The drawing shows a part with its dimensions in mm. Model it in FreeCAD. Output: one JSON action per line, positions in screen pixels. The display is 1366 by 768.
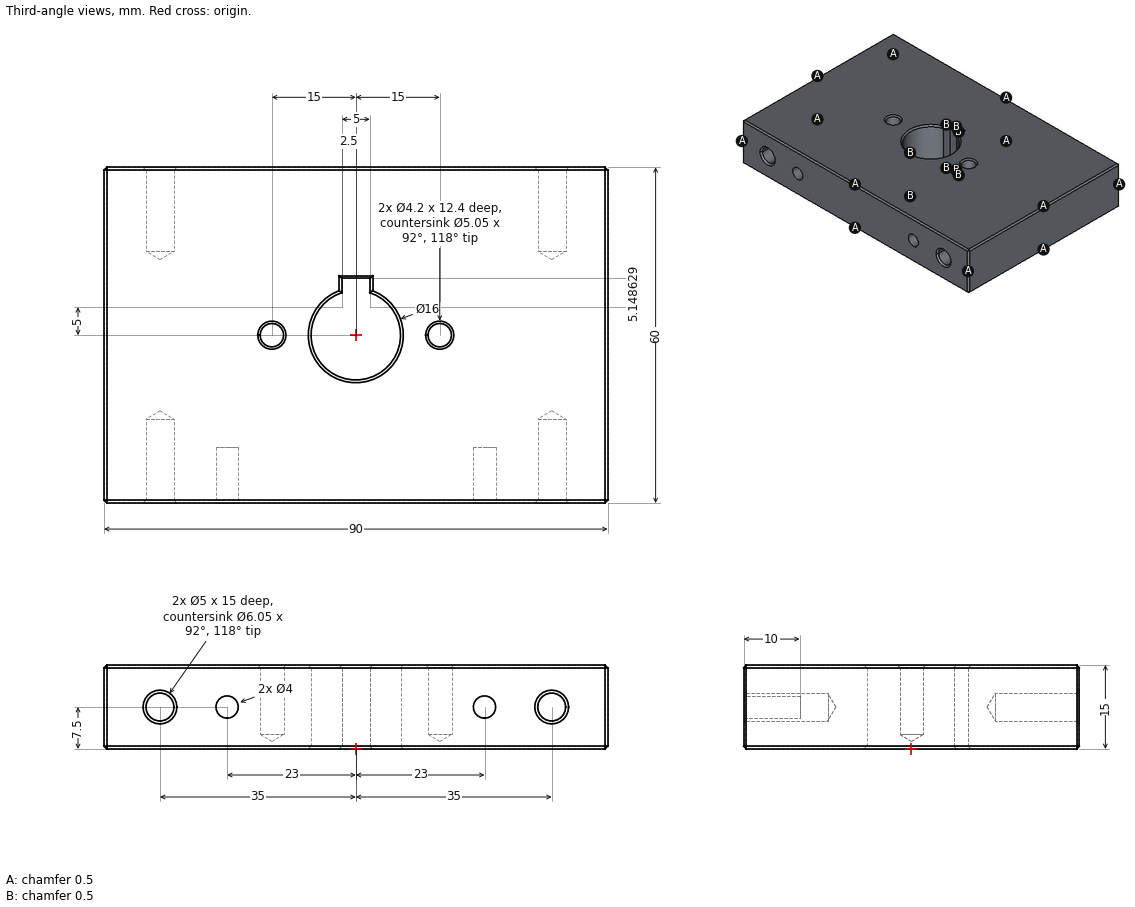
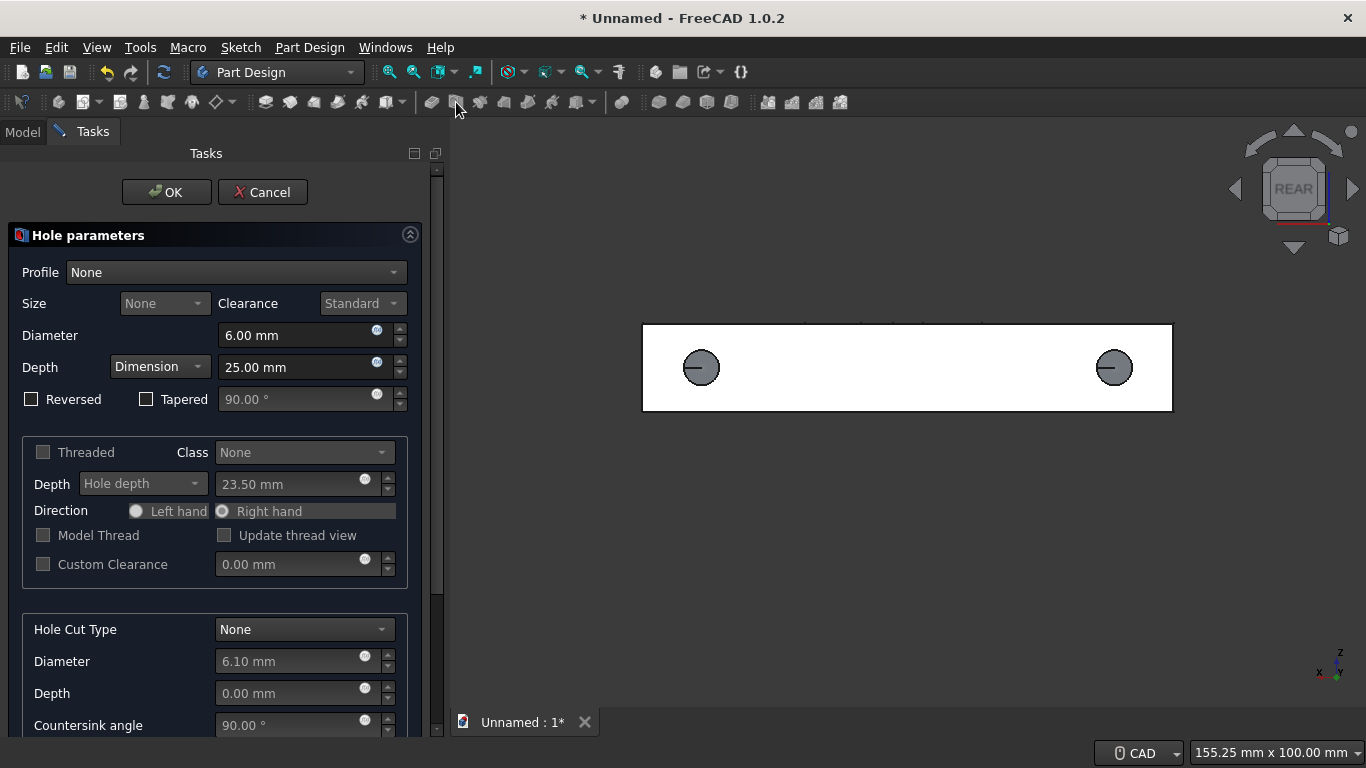
{"action": "triple_click", "coordinate": [305, 335]}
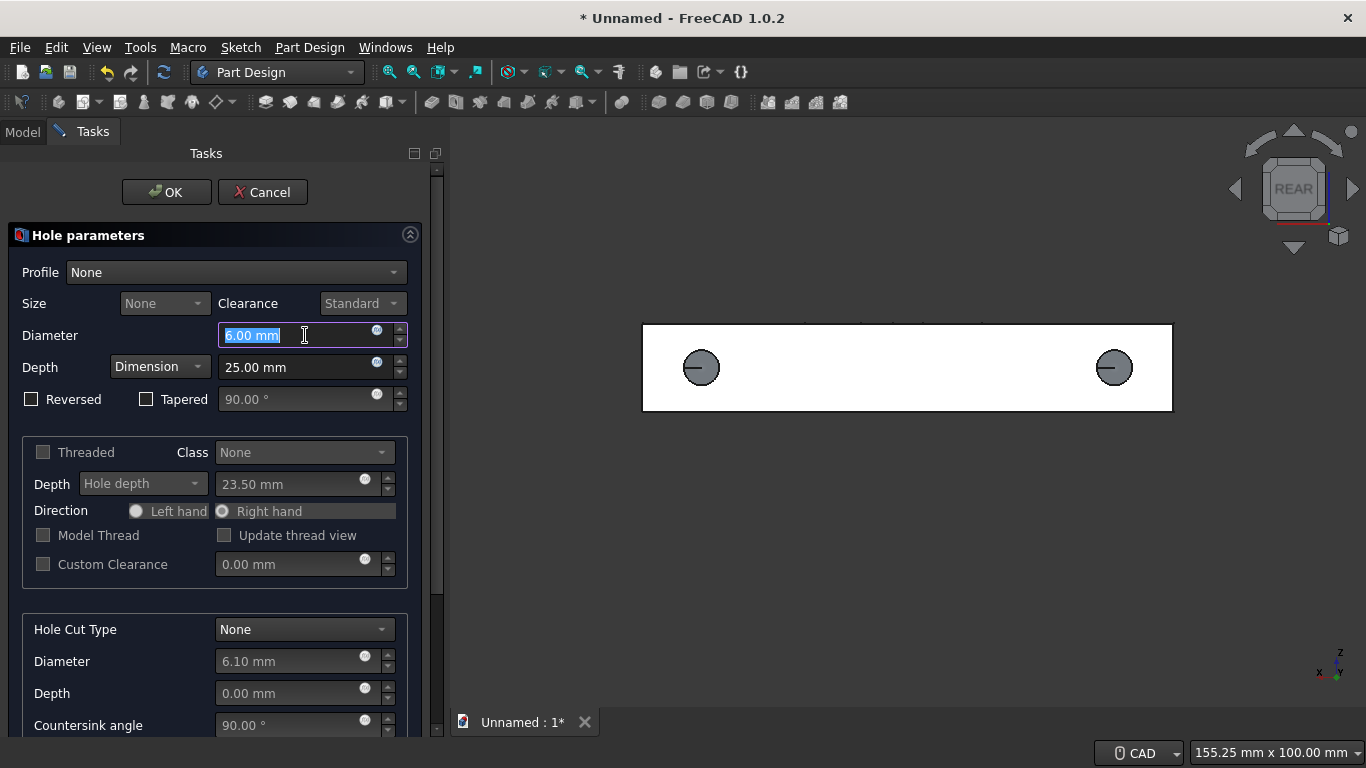
{"action": "type", "text": "5"}
{"action": "key", "text": "Tab"}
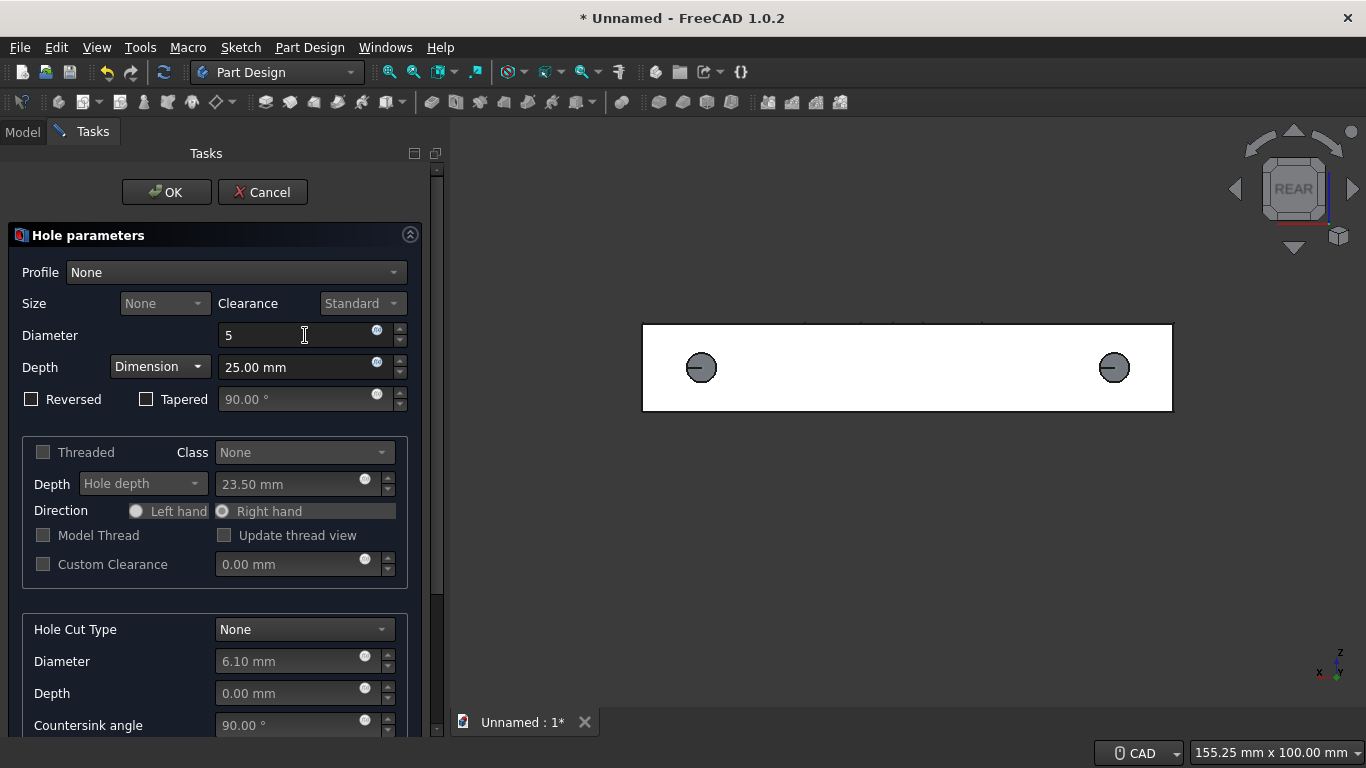
{"action": "triple_click", "coordinate": [305, 367]}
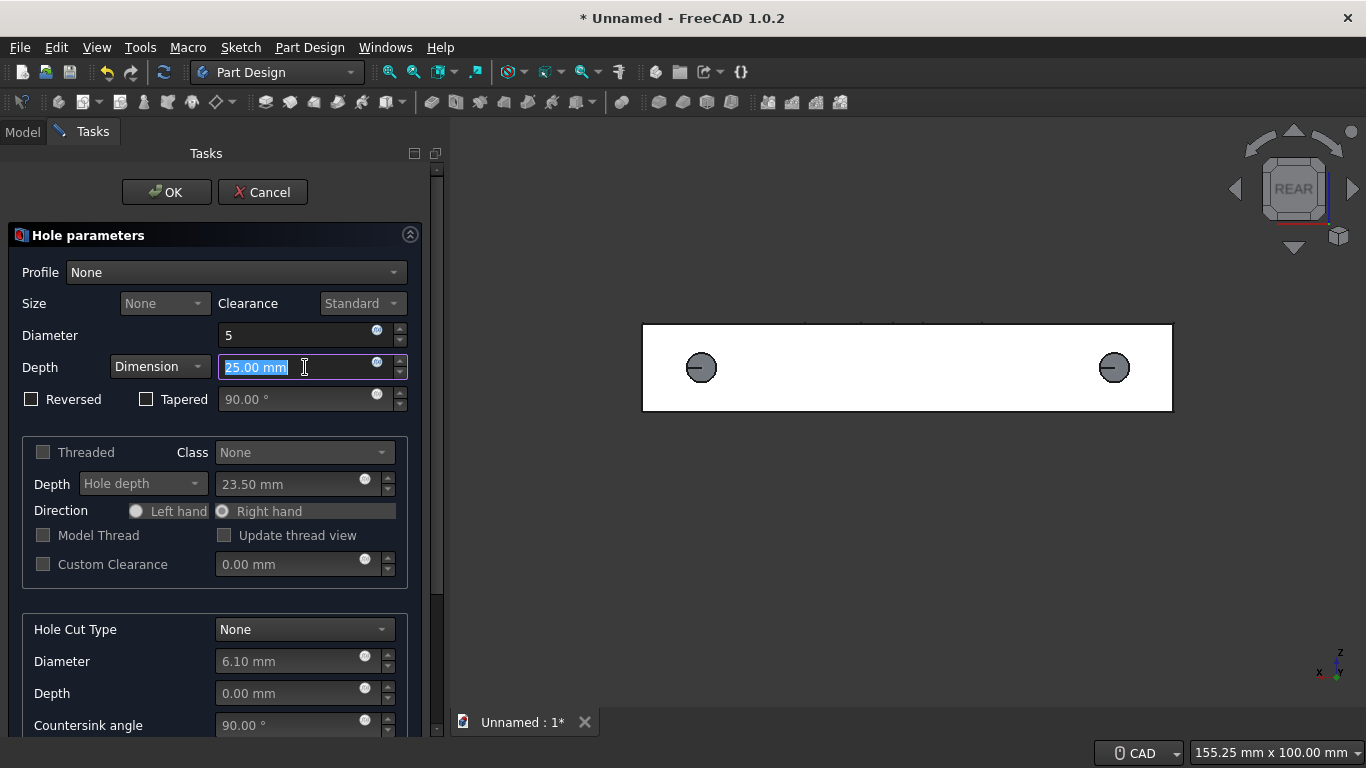
{"action": "type", "text": "15"}
{"action": "key", "text": "Tab"}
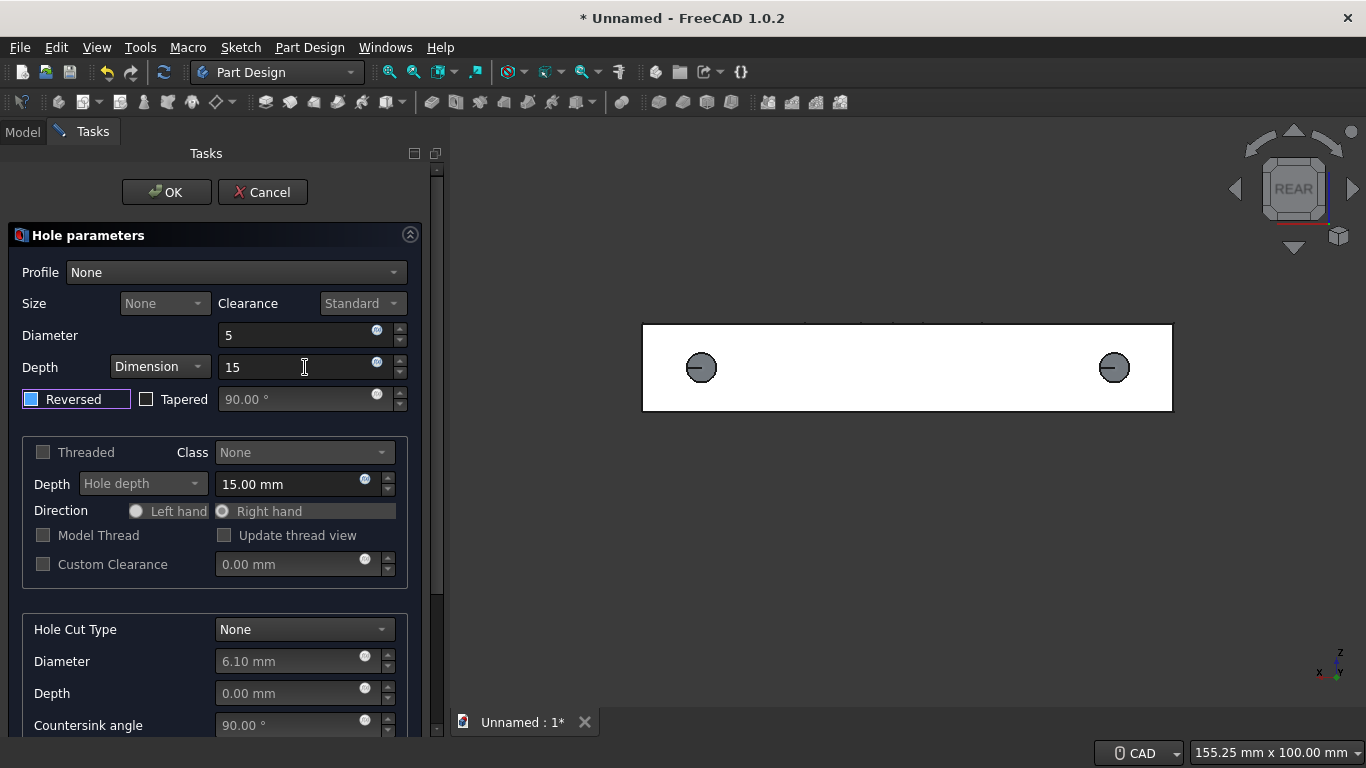
{"action": "left_click", "coordinate": [306, 630]}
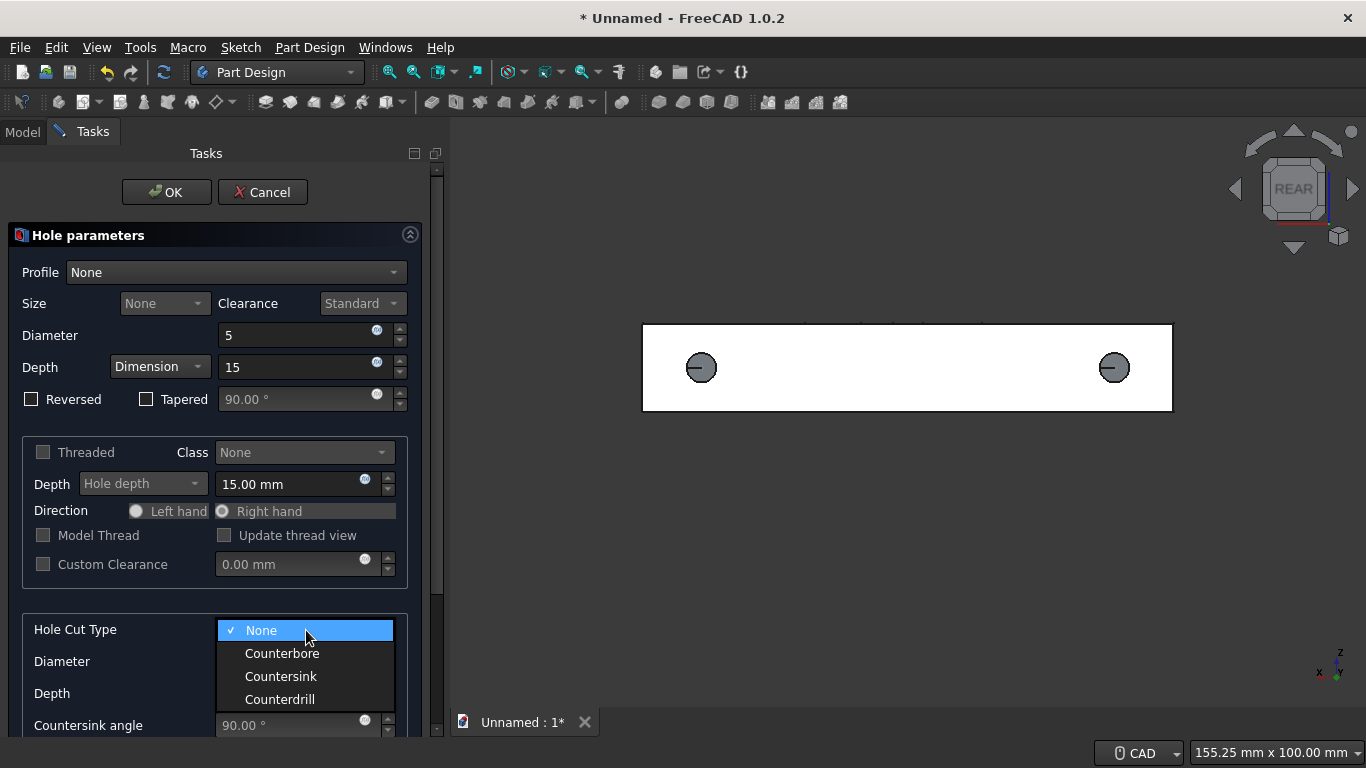
{"action": "left_click", "coordinate": [304, 676]}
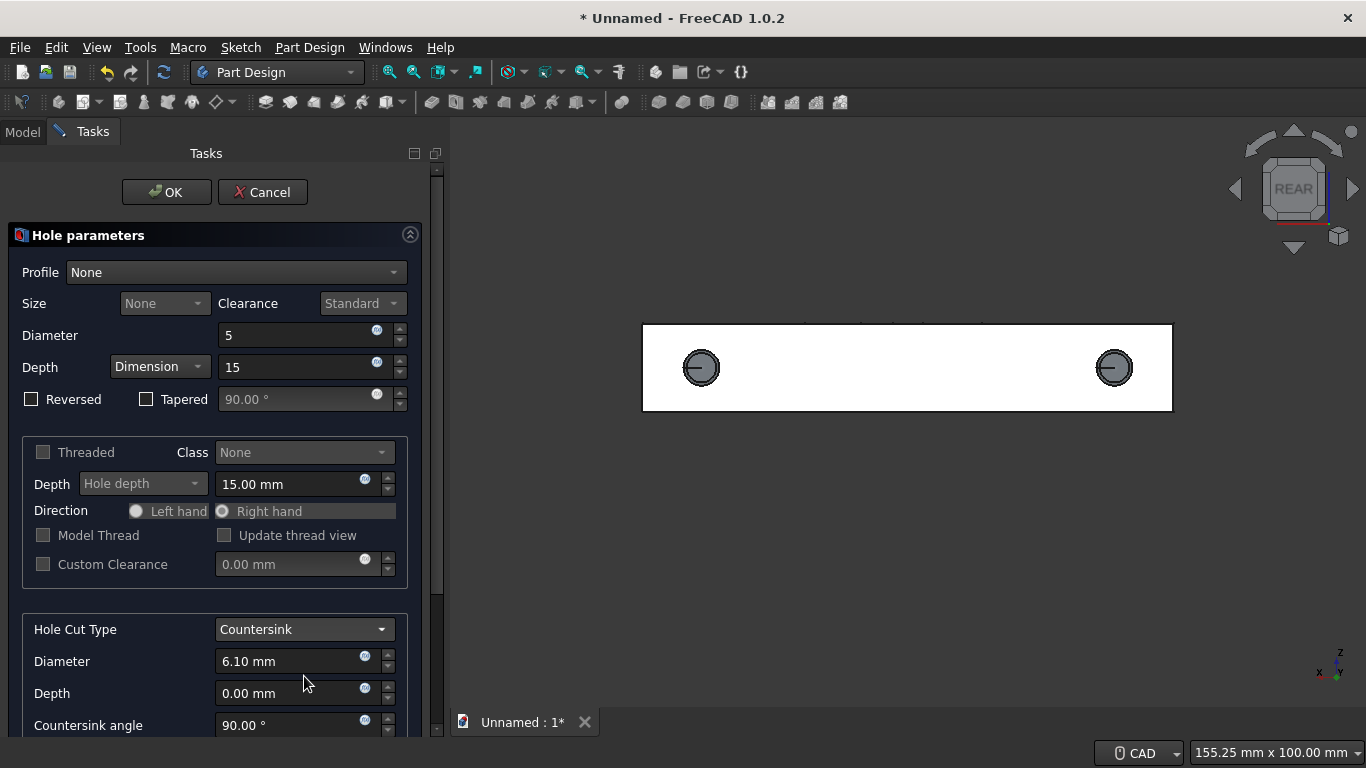
{"action": "scroll", "coordinate": [437, 450], "scroll_direction": "down", "scroll_amount": 2}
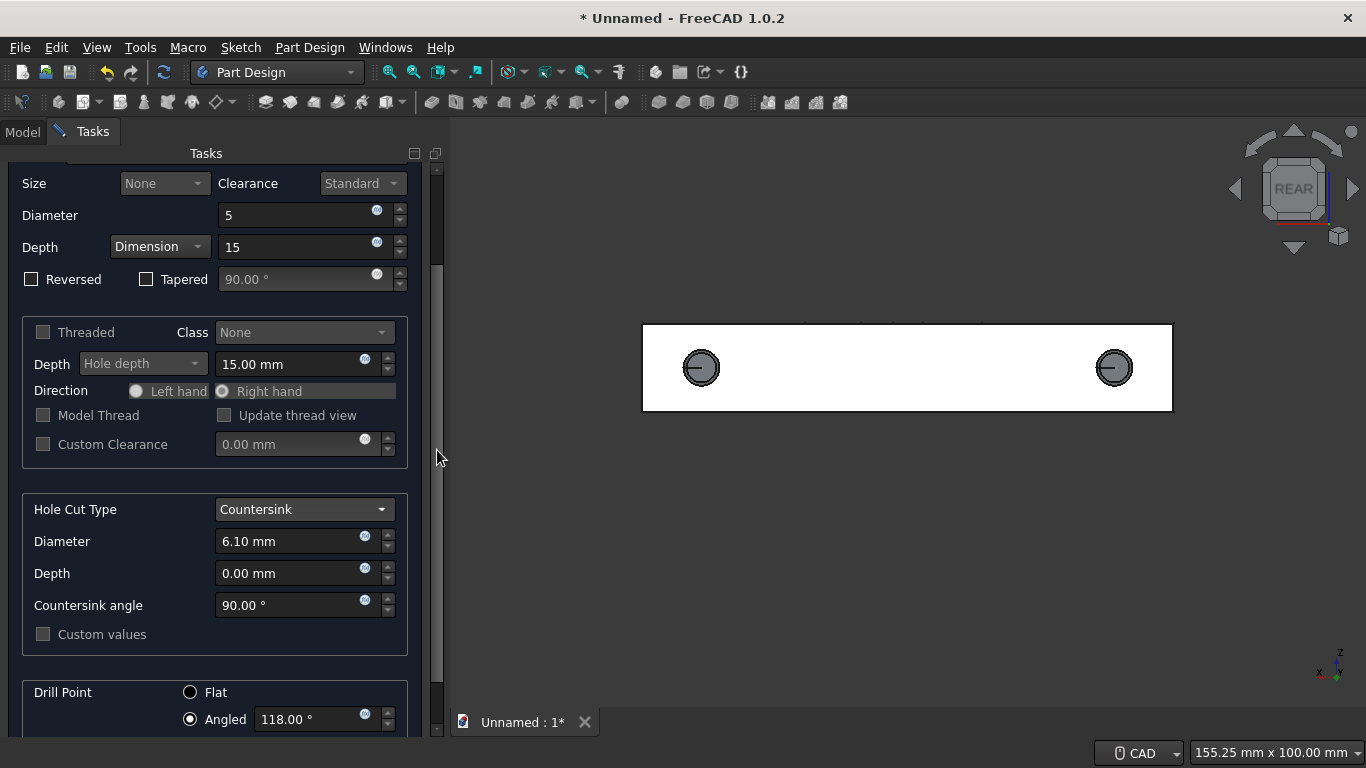
{"action": "triple_click", "coordinate": [298, 605]}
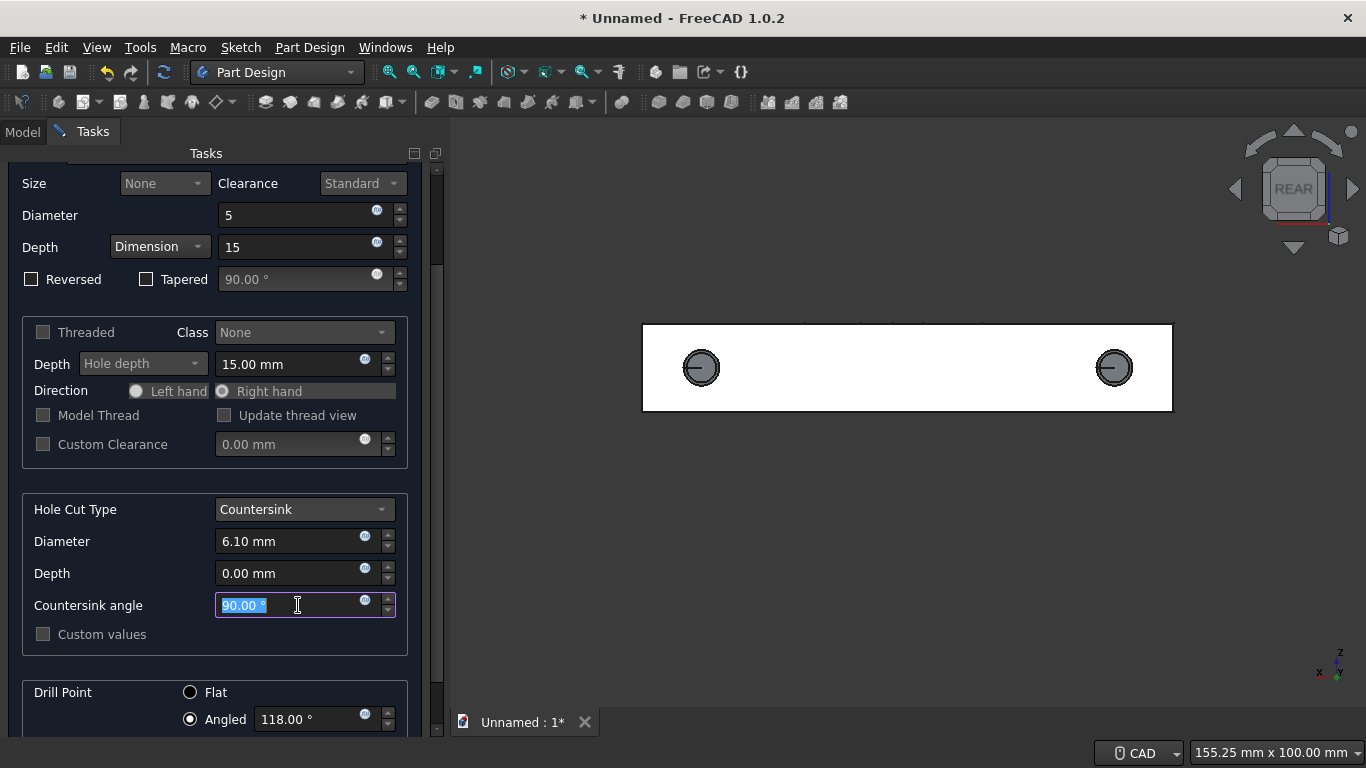
{"action": "type", "text": "92"}
{"action": "key", "text": "Tab"}